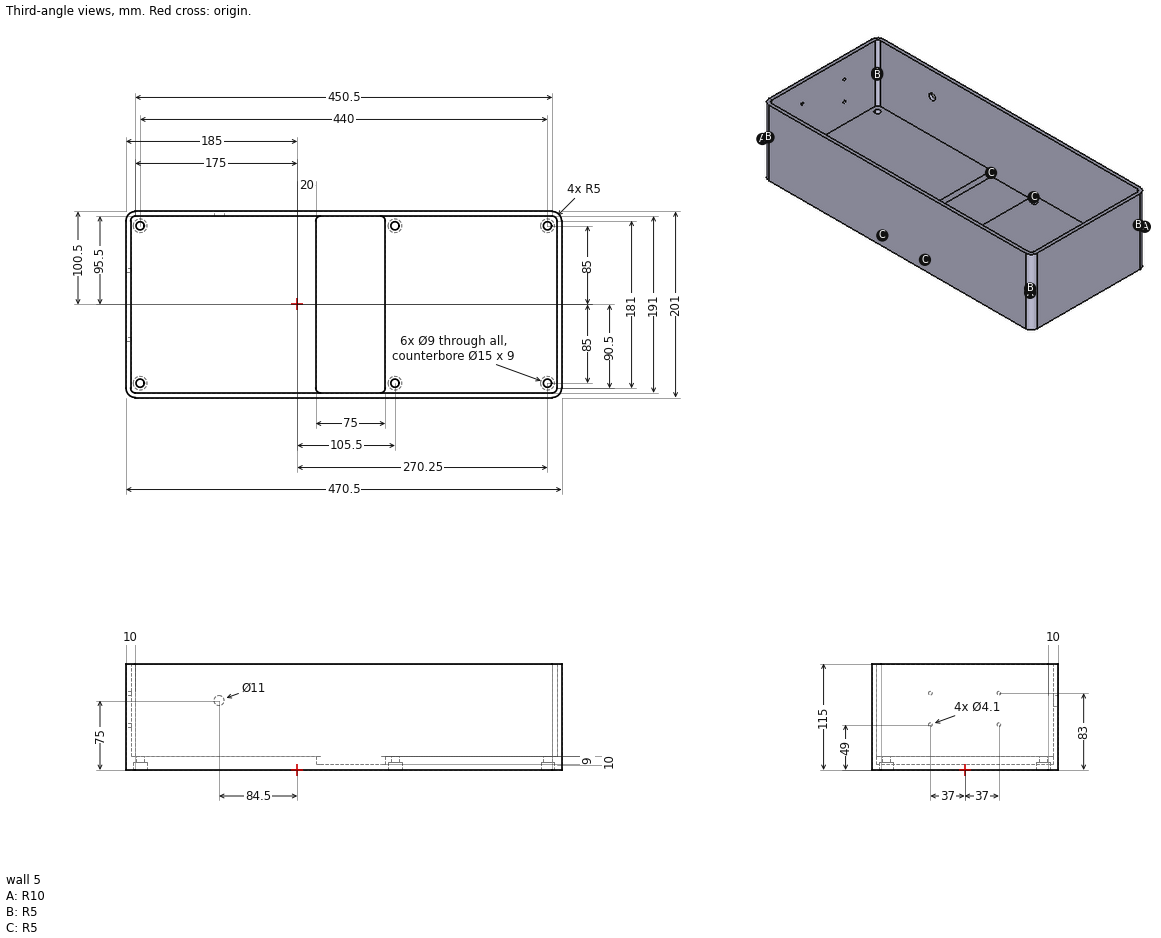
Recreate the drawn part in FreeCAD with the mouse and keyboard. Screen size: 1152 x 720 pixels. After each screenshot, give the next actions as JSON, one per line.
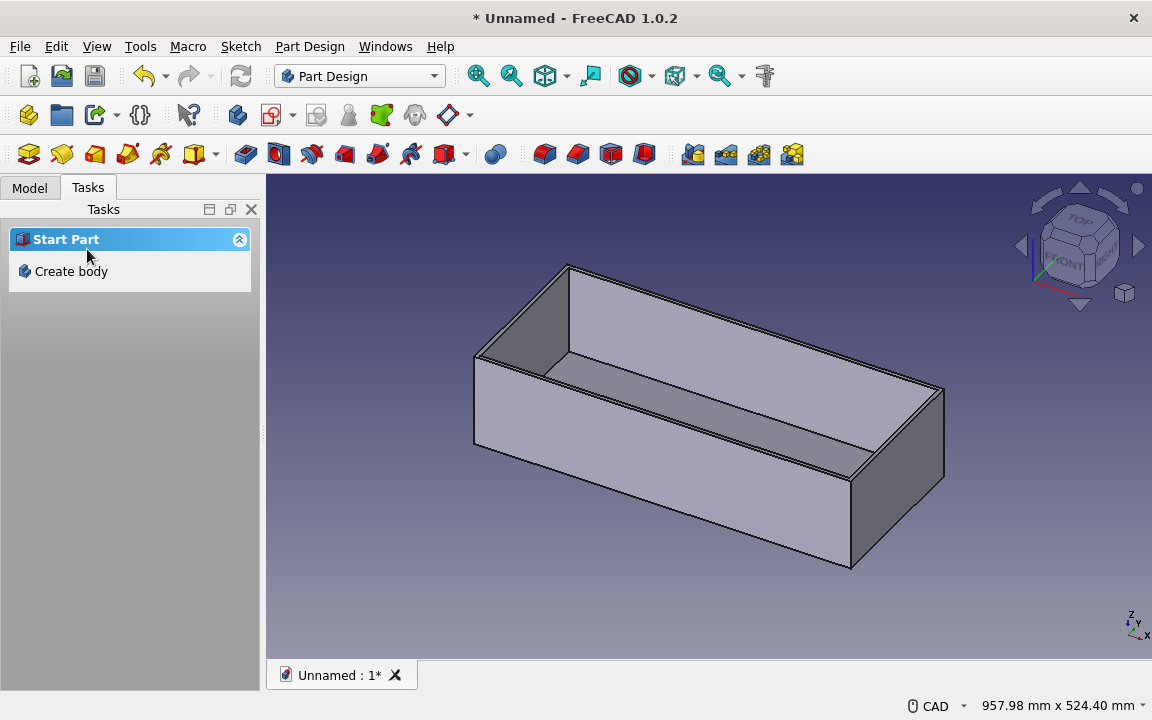
{"action": "key", "text": "4"}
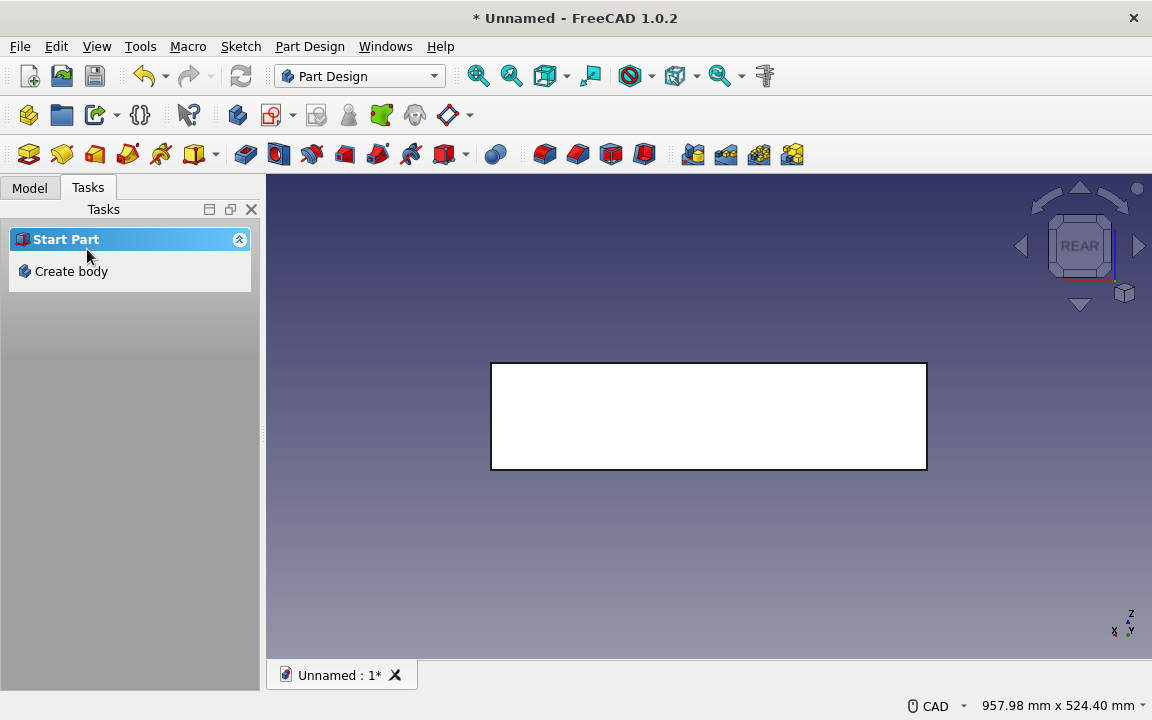
{"action": "left_click", "coordinate": [585, 415]}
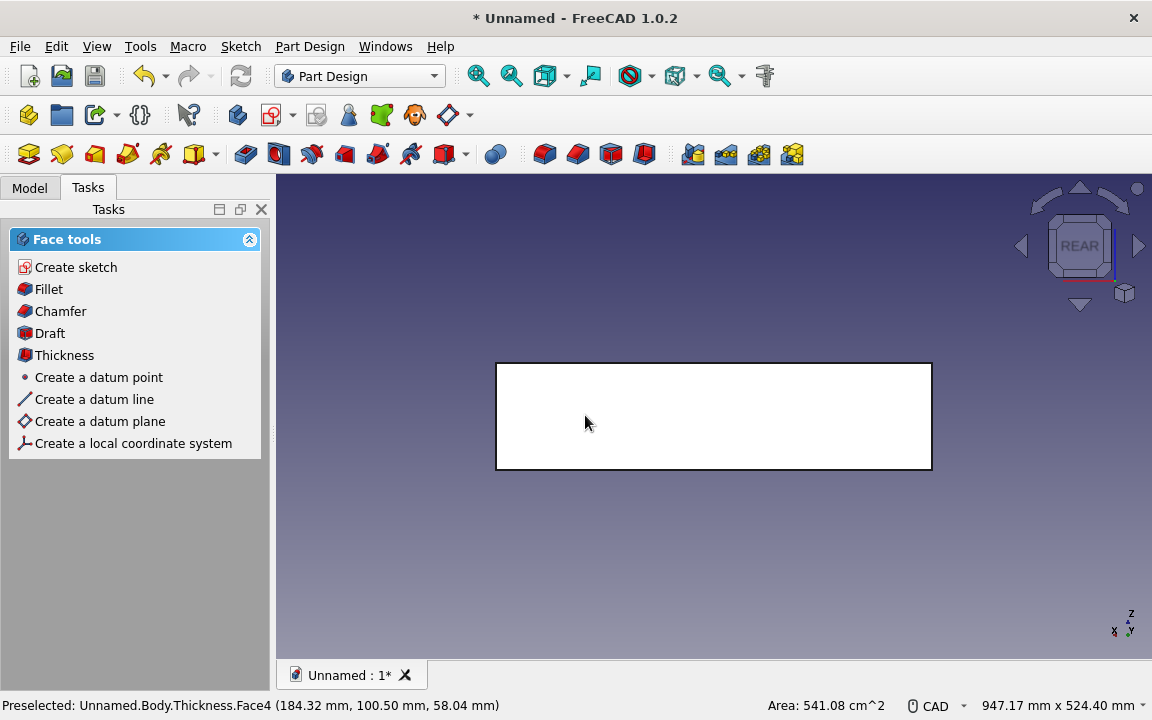
{"action": "left_click", "coordinate": [270, 116]}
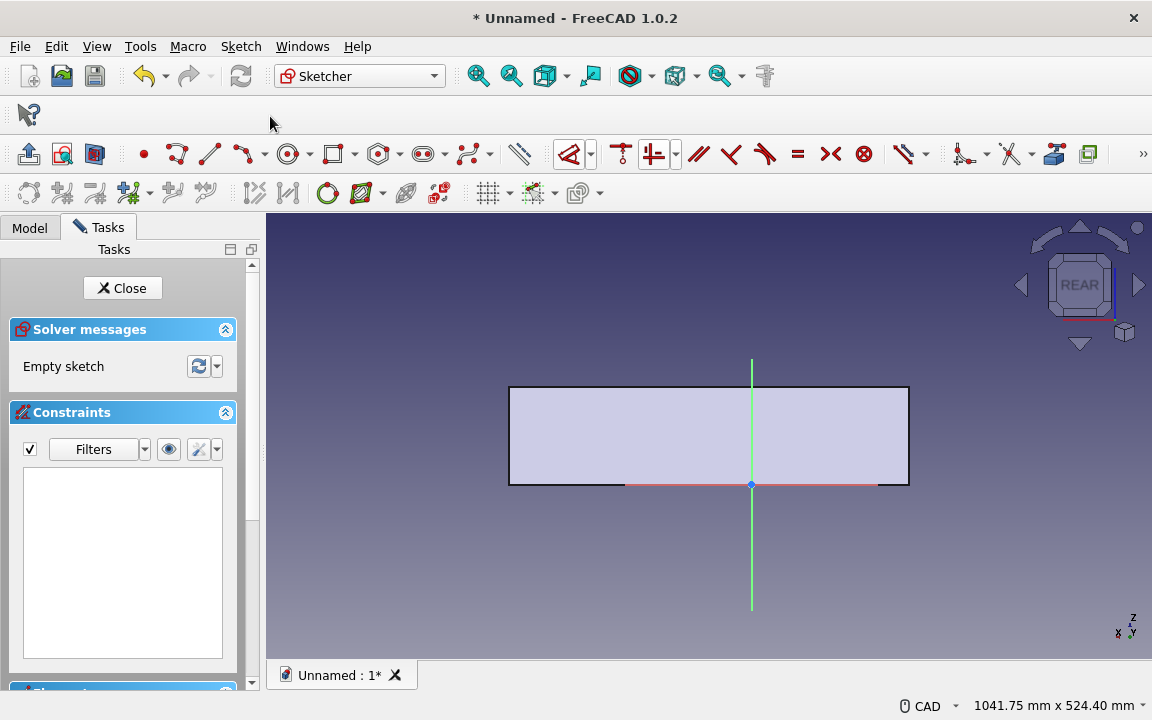
{"action": "scroll", "coordinate": [833, 420], "scroll_direction": "up", "scroll_amount": 15}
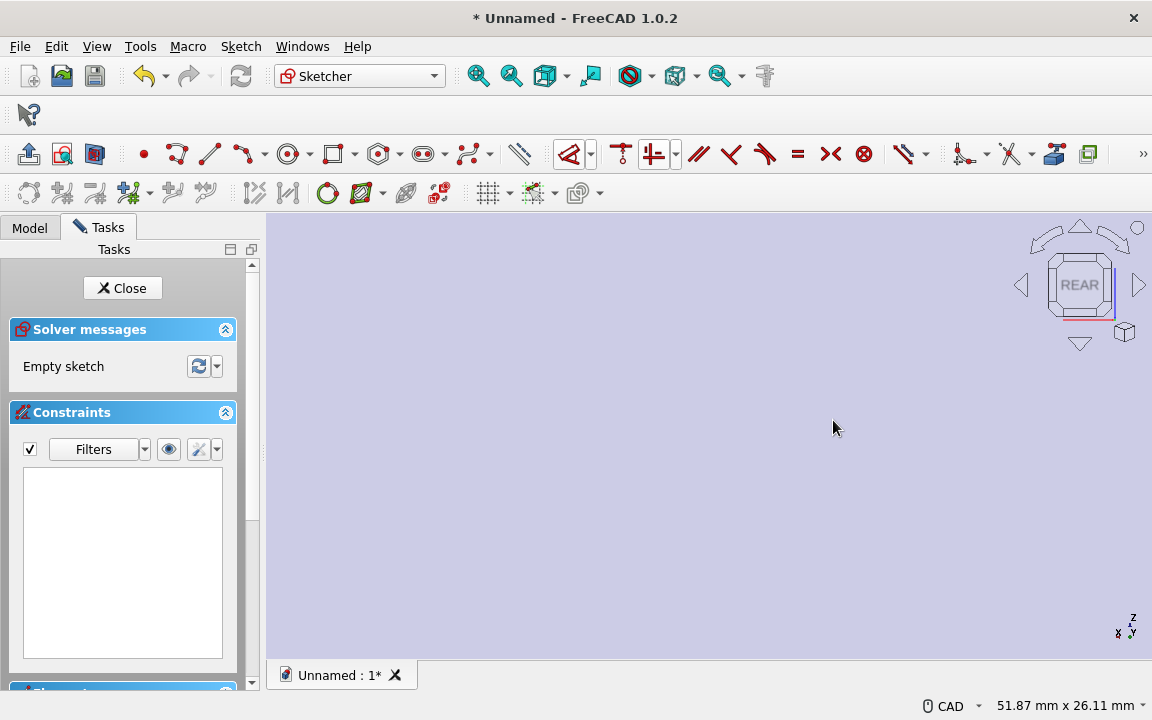
{"action": "scroll", "coordinate": [615, 429], "scroll_direction": "up", "scroll_amount": 2}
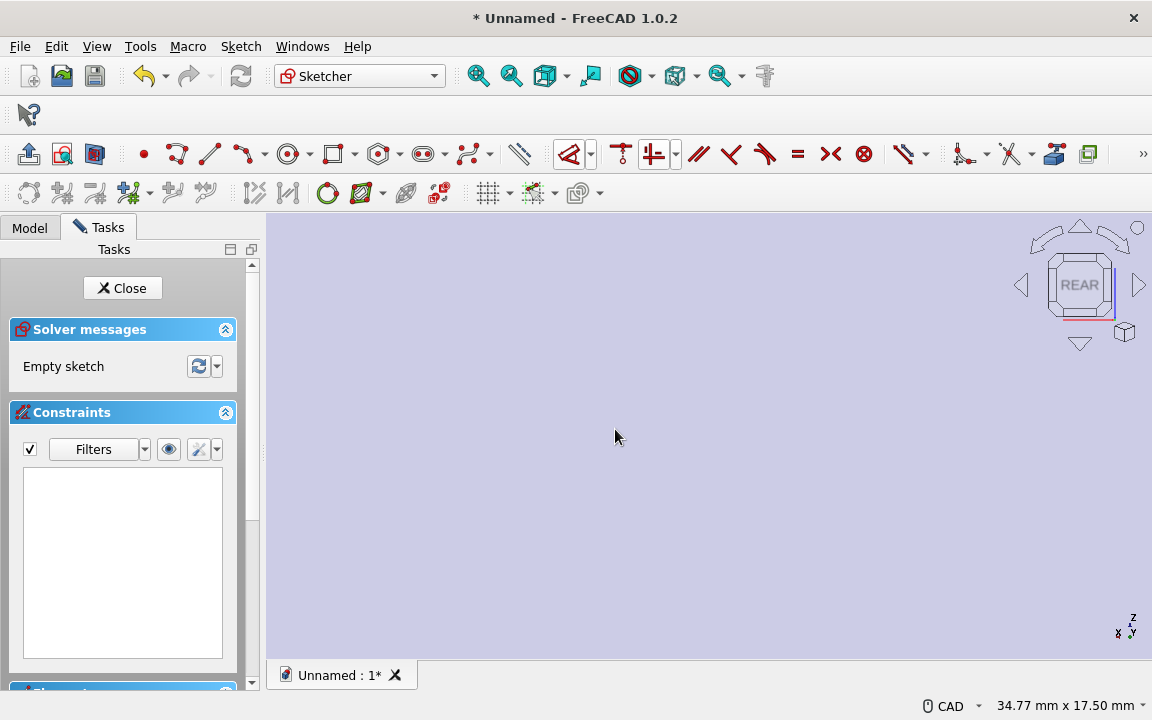
{"action": "key", "text": "g c"}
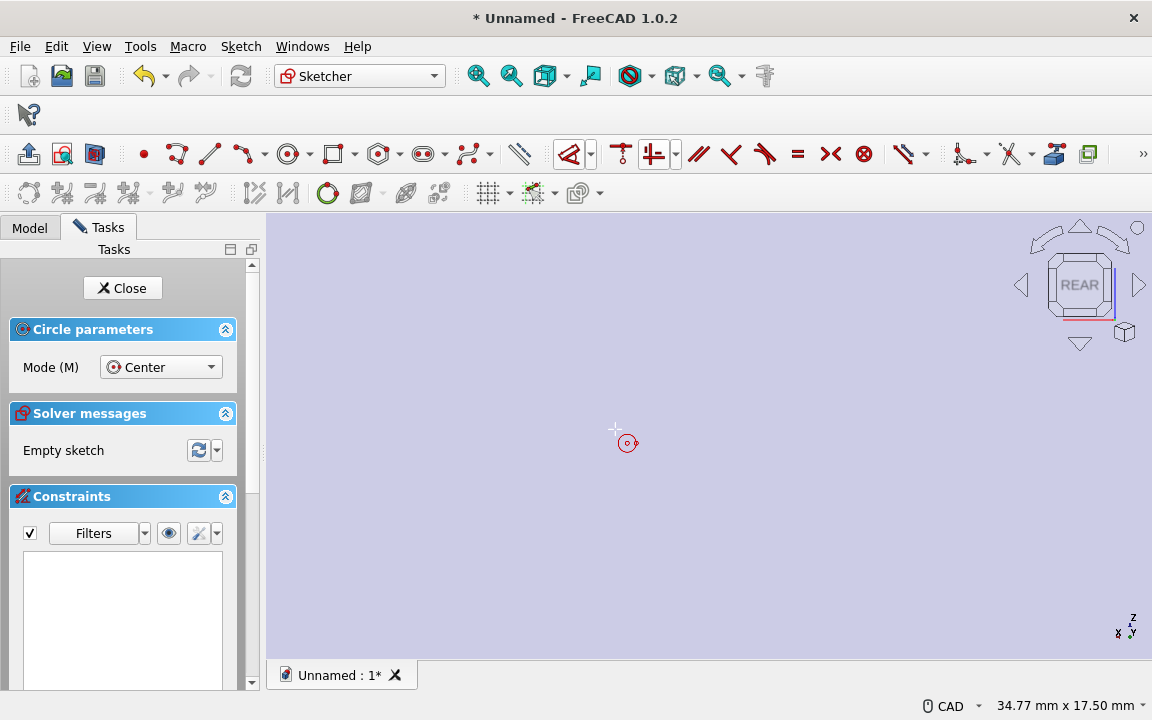
{"action": "left_click", "coordinate": [640, 436]}
{"action": "mouse_move", "coordinate": [739, 336]}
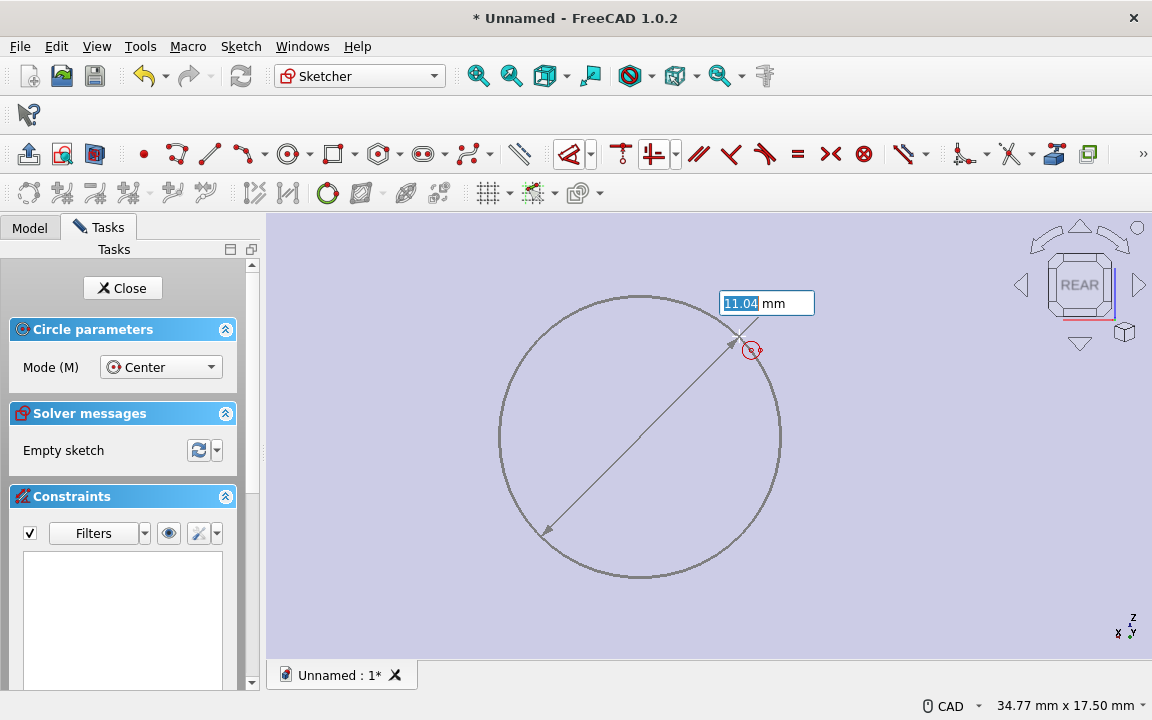
{"action": "type", "text": "11"}
{"action": "key", "text": "Return"}
{"action": "key", "text": "Escape"}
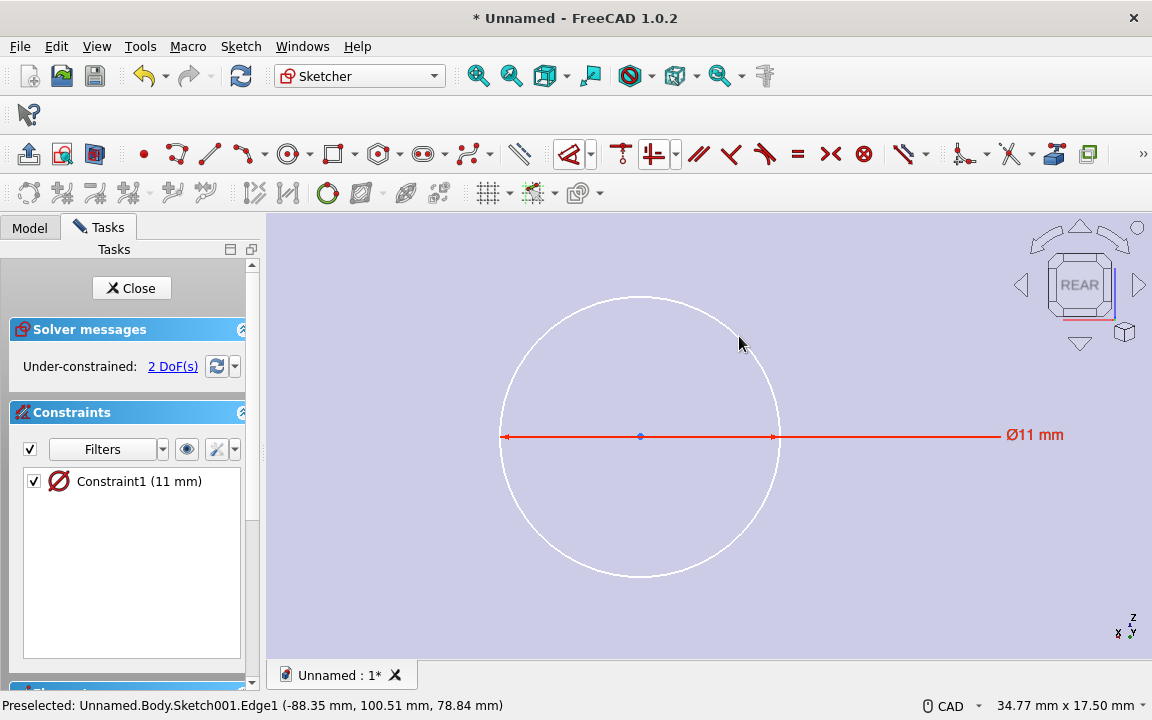
{"action": "key", "text": "d"}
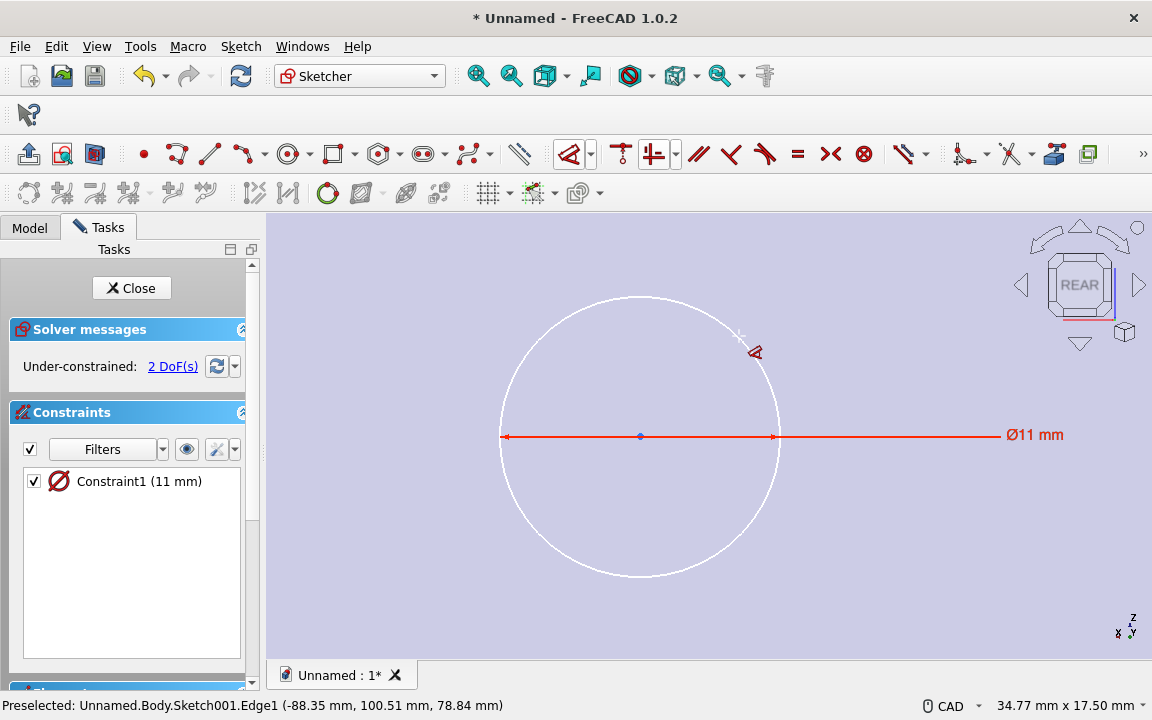
{"action": "left_click", "coordinate": [640, 437]}
{"action": "left_click", "coordinate": [674, 534]}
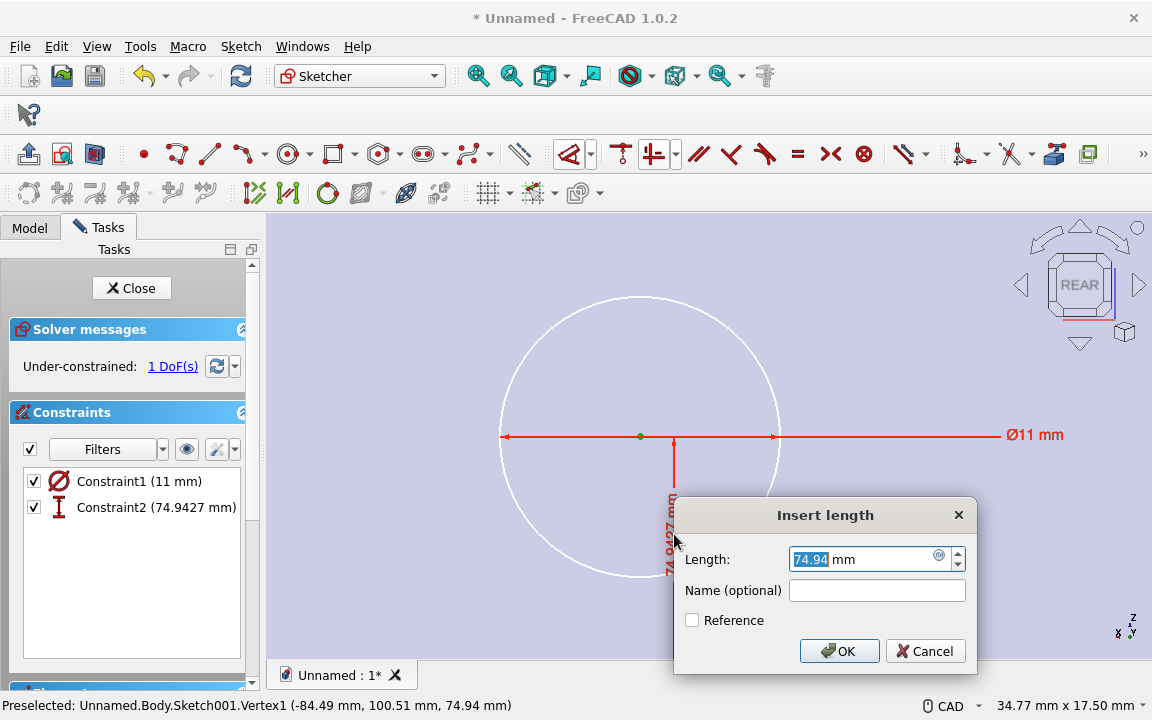
{"action": "type", "text": "75"}
{"action": "key", "text": "Return"}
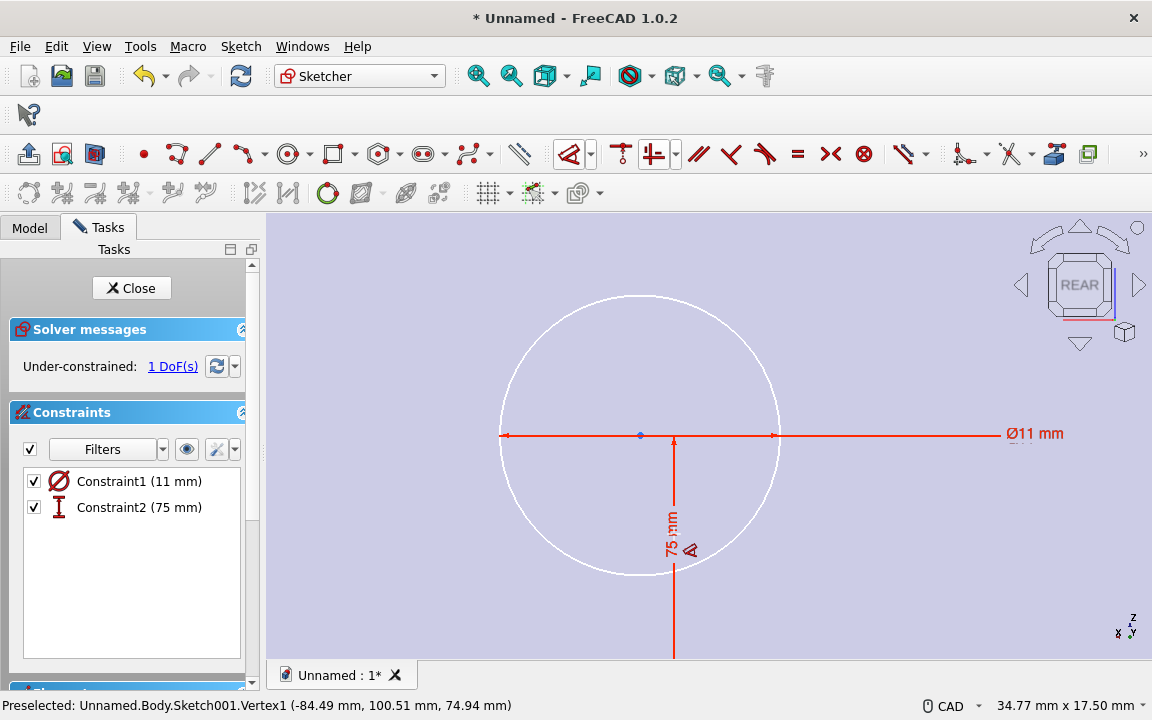
{"action": "left_click", "coordinate": [640, 436]}
{"action": "left_click", "coordinate": [467, 402]}